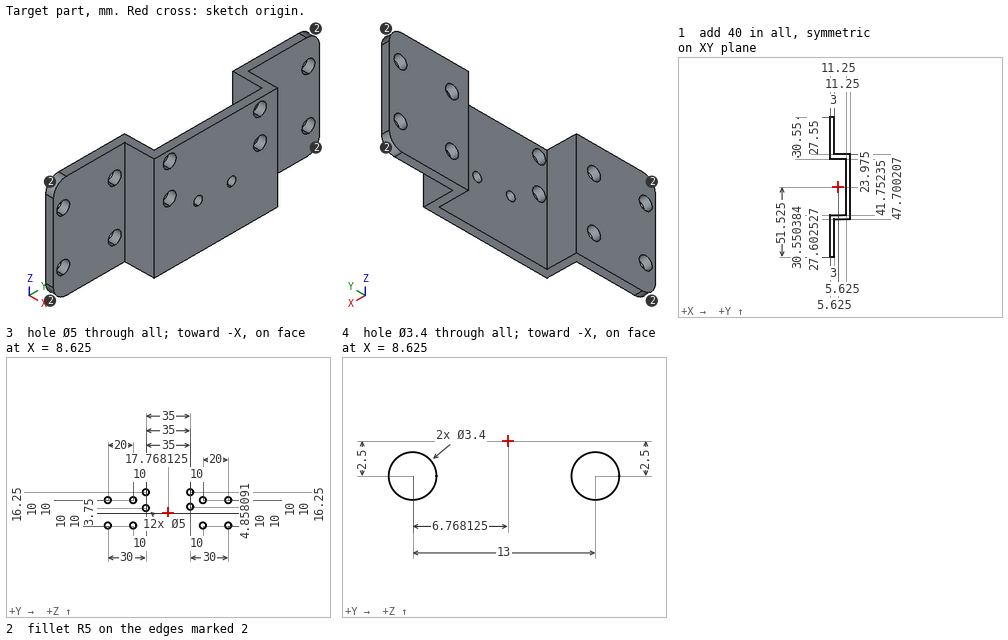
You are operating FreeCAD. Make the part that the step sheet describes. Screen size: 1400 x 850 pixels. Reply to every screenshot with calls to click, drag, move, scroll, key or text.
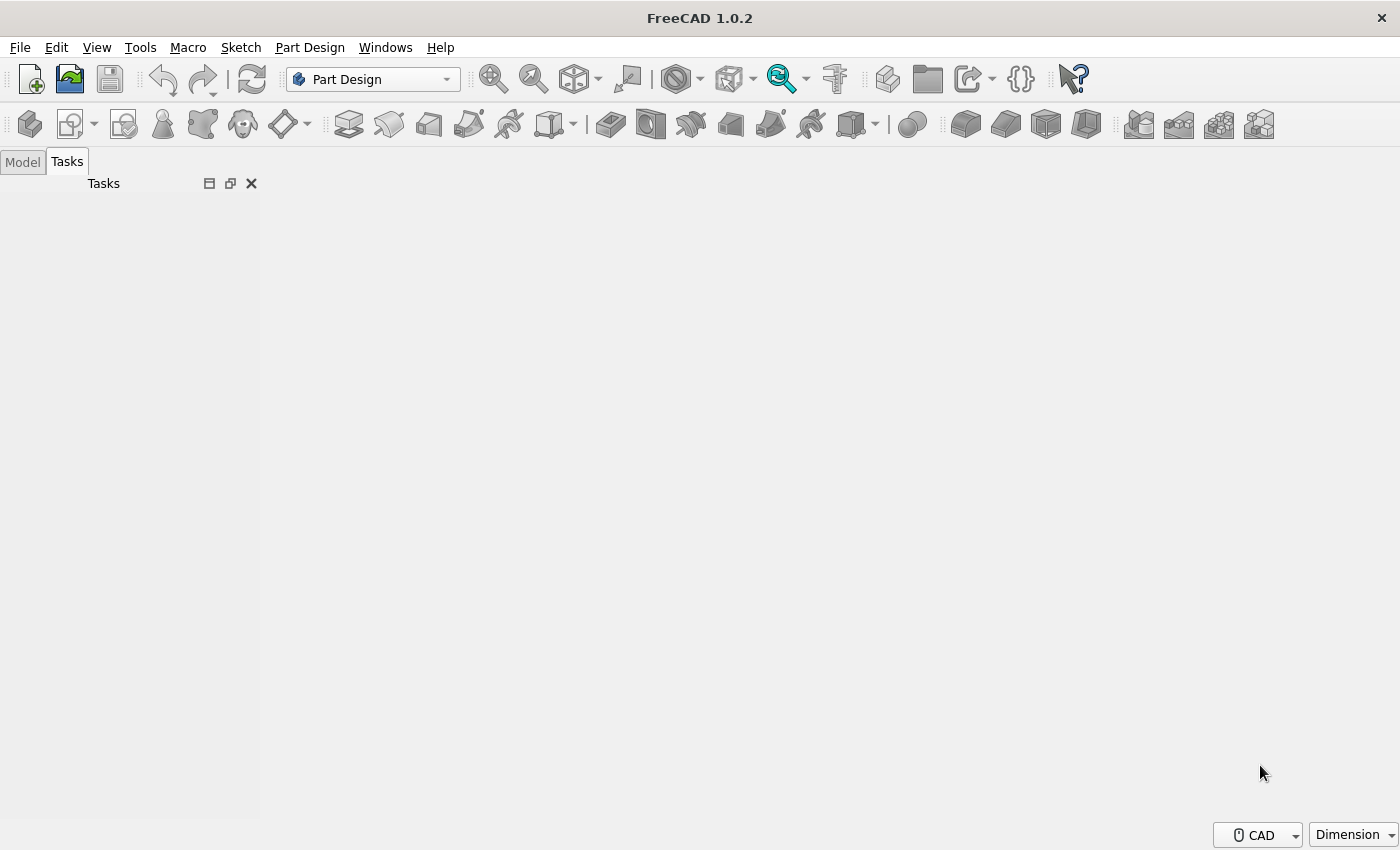
key(ctrl+n)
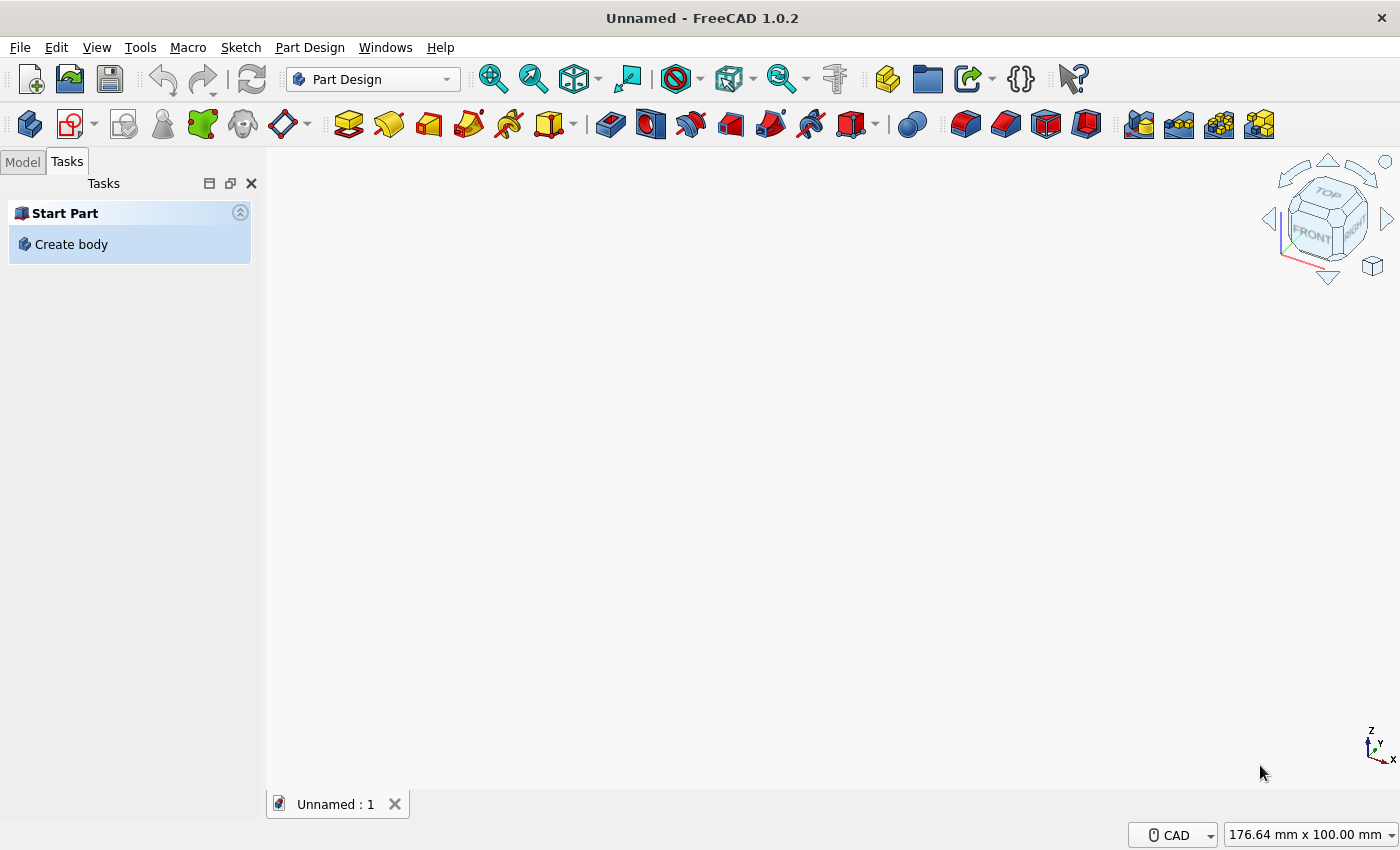
click(70, 124)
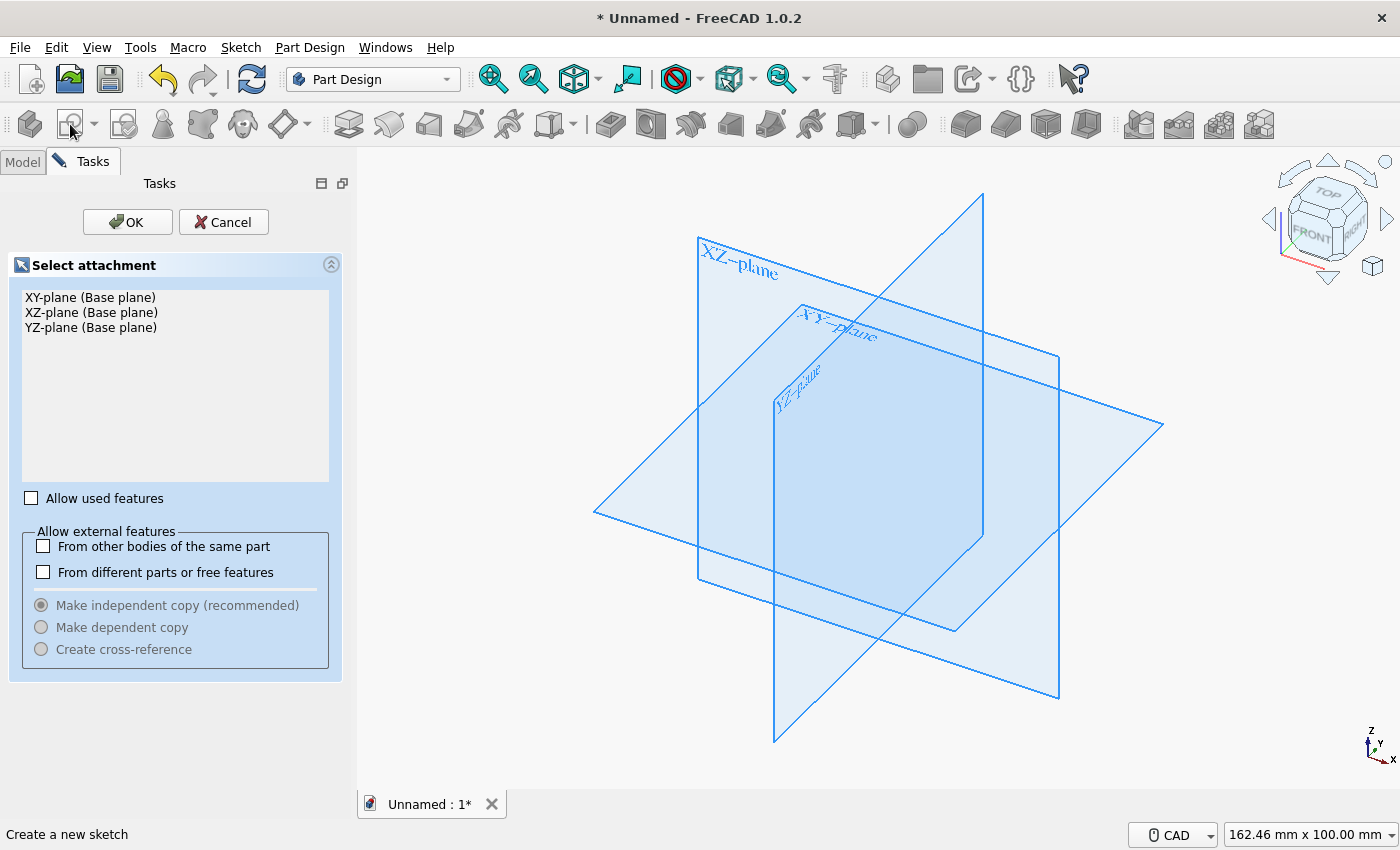
click(82, 298)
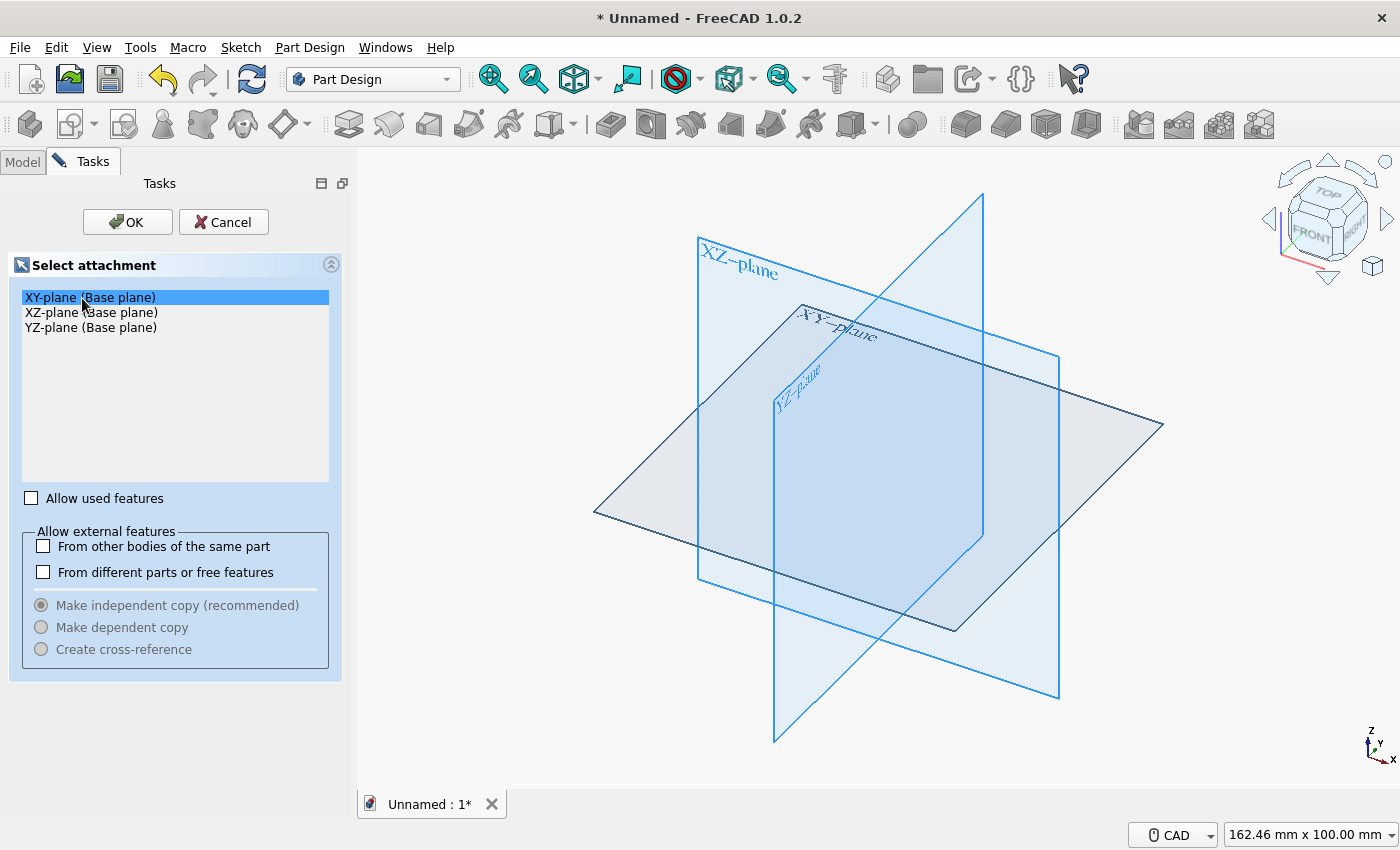
click(128, 222)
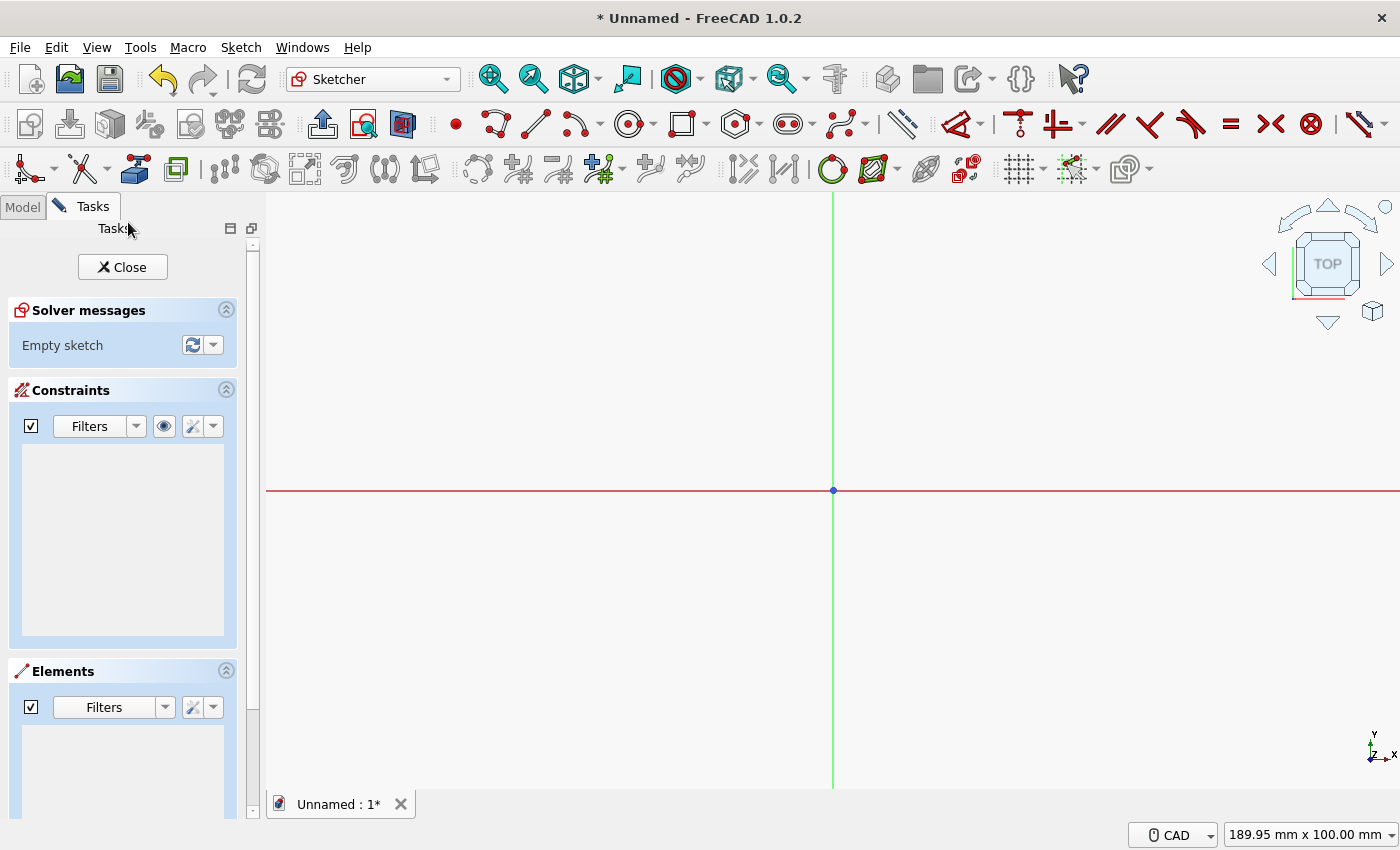
scroll(607, 490, down, 2)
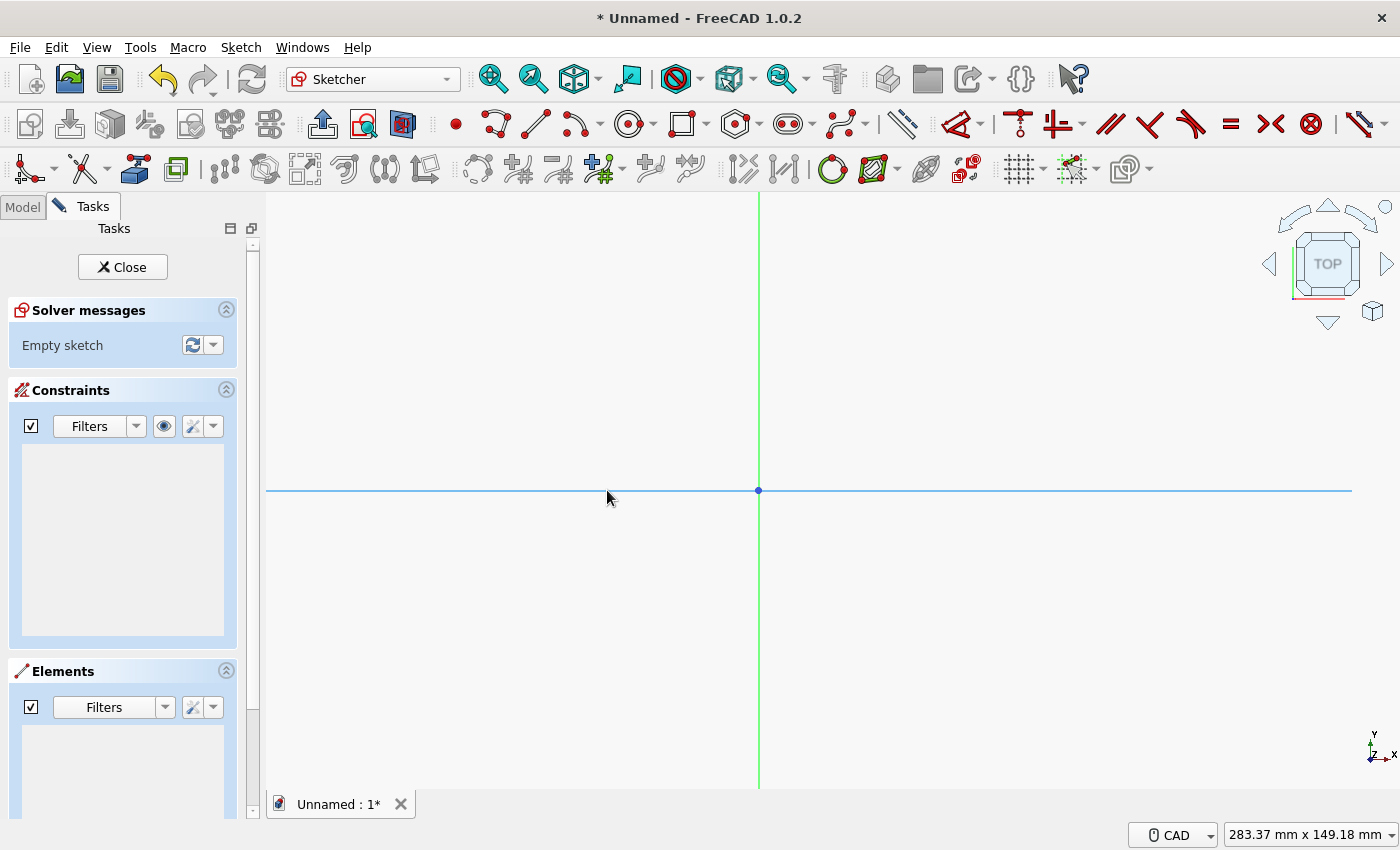
click(496, 124)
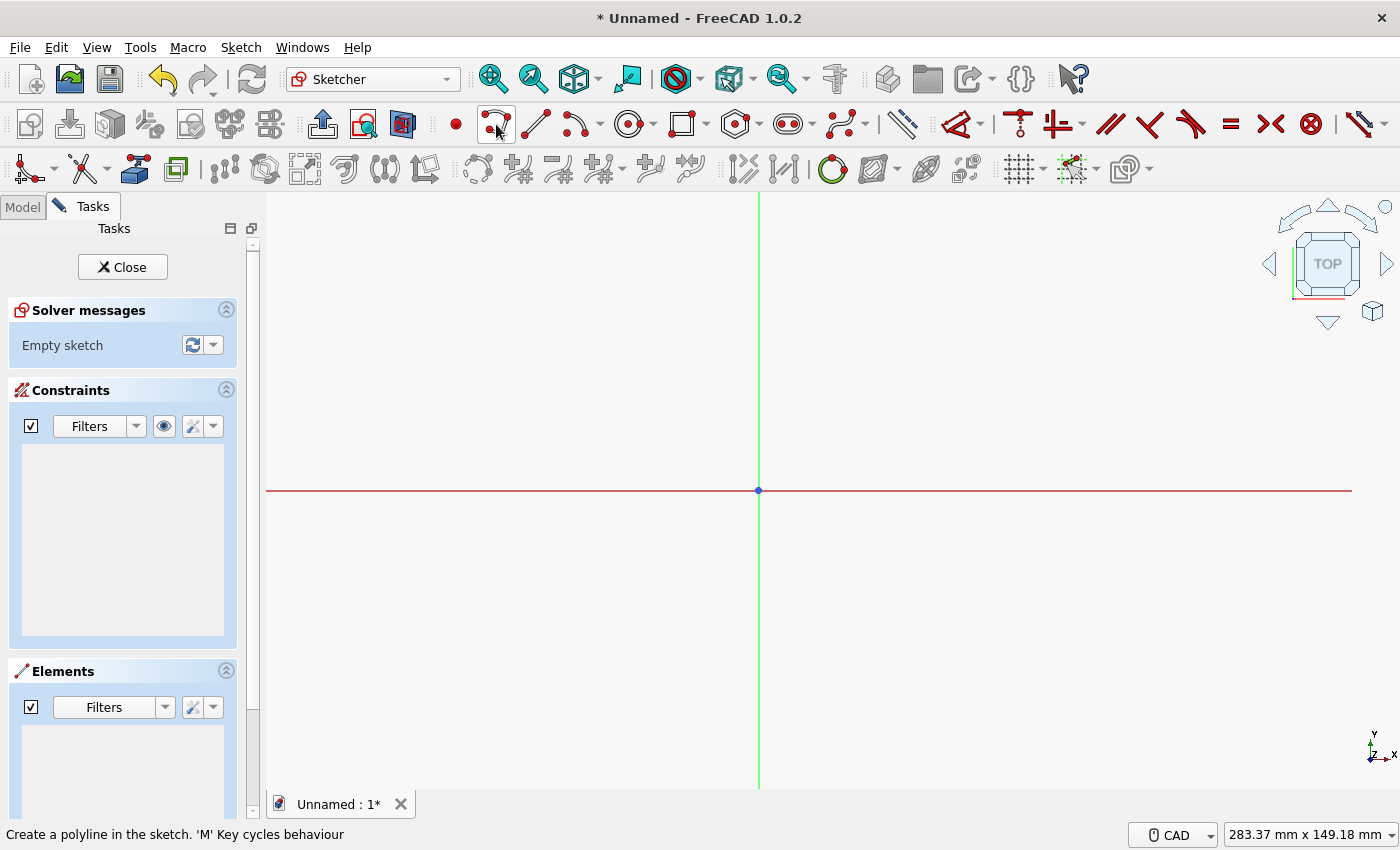
click(781, 574)
click(736, 578)
click(736, 697)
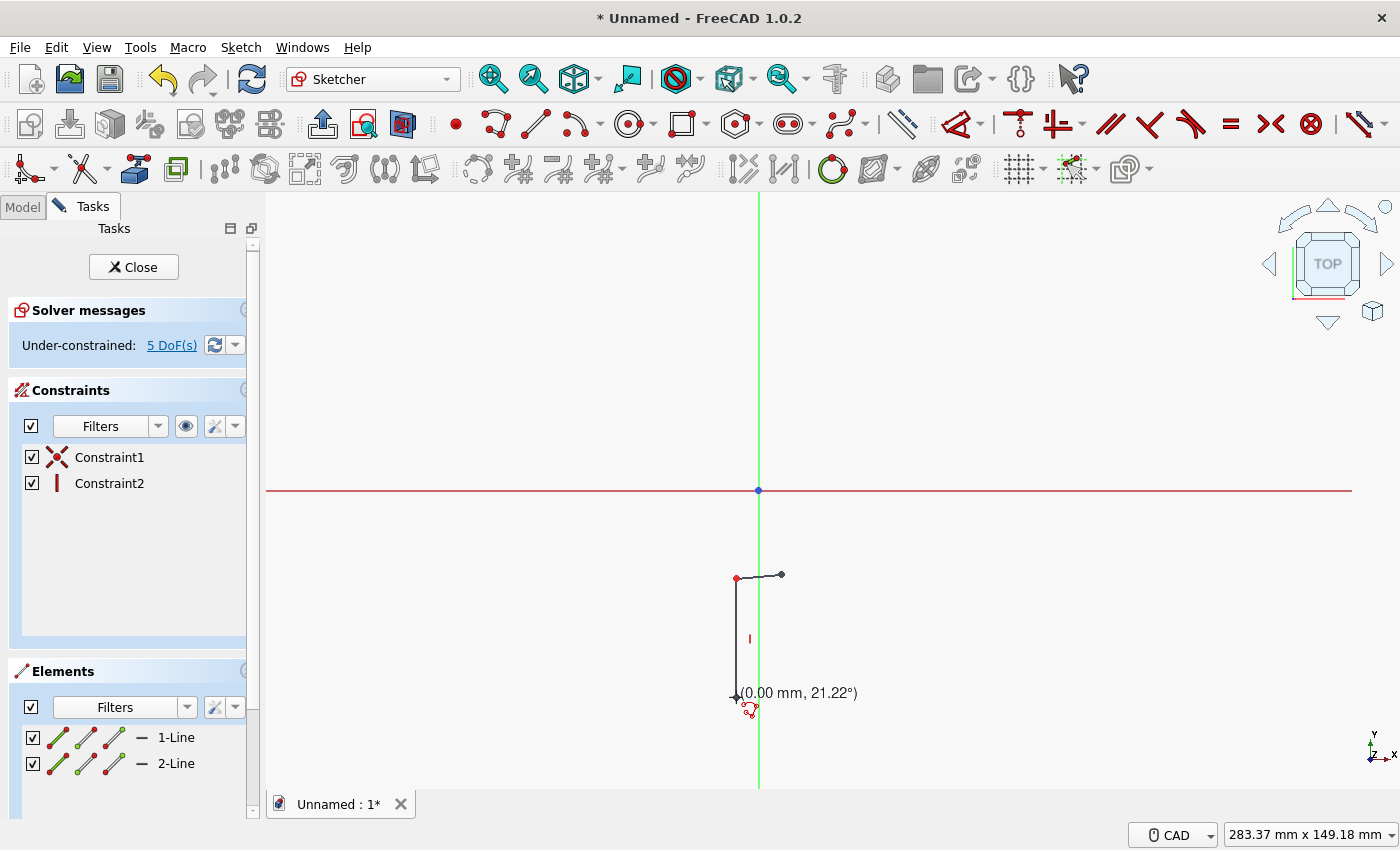
scroll(748, 697, up, 3)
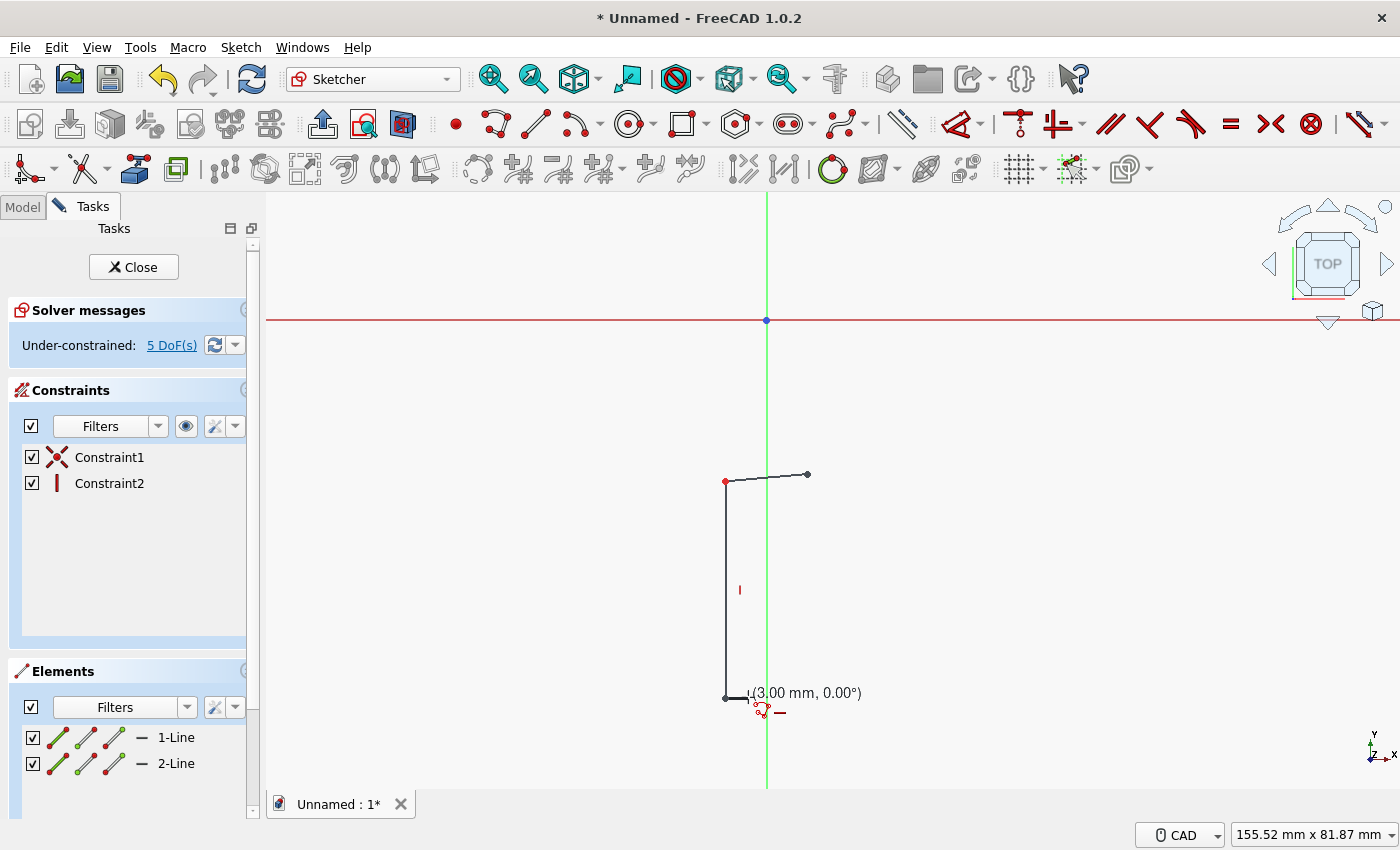
click(748, 696)
click(748, 494)
click(830, 489)